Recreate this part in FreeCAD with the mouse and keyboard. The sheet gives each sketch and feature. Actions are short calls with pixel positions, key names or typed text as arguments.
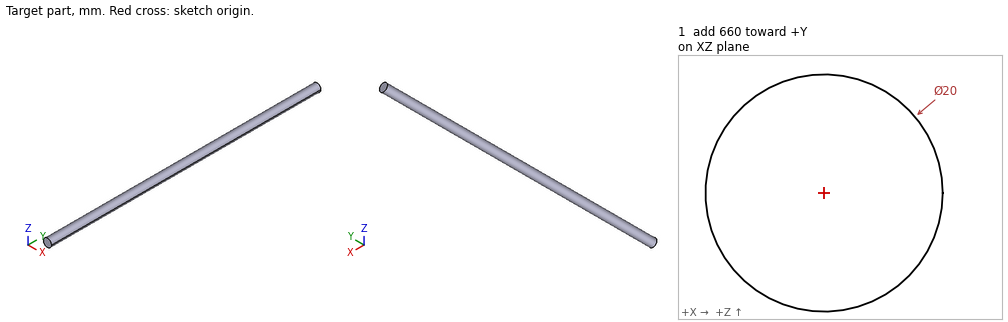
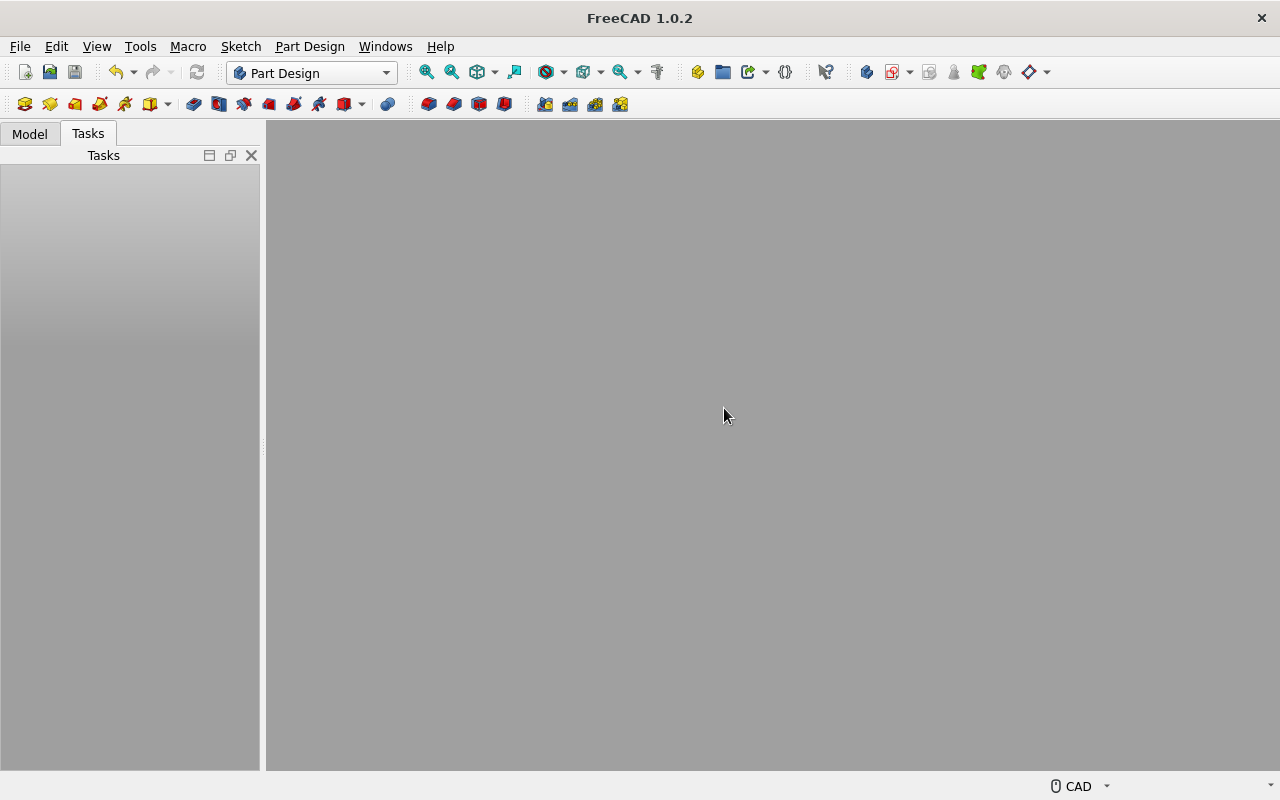
key(ctrl+n)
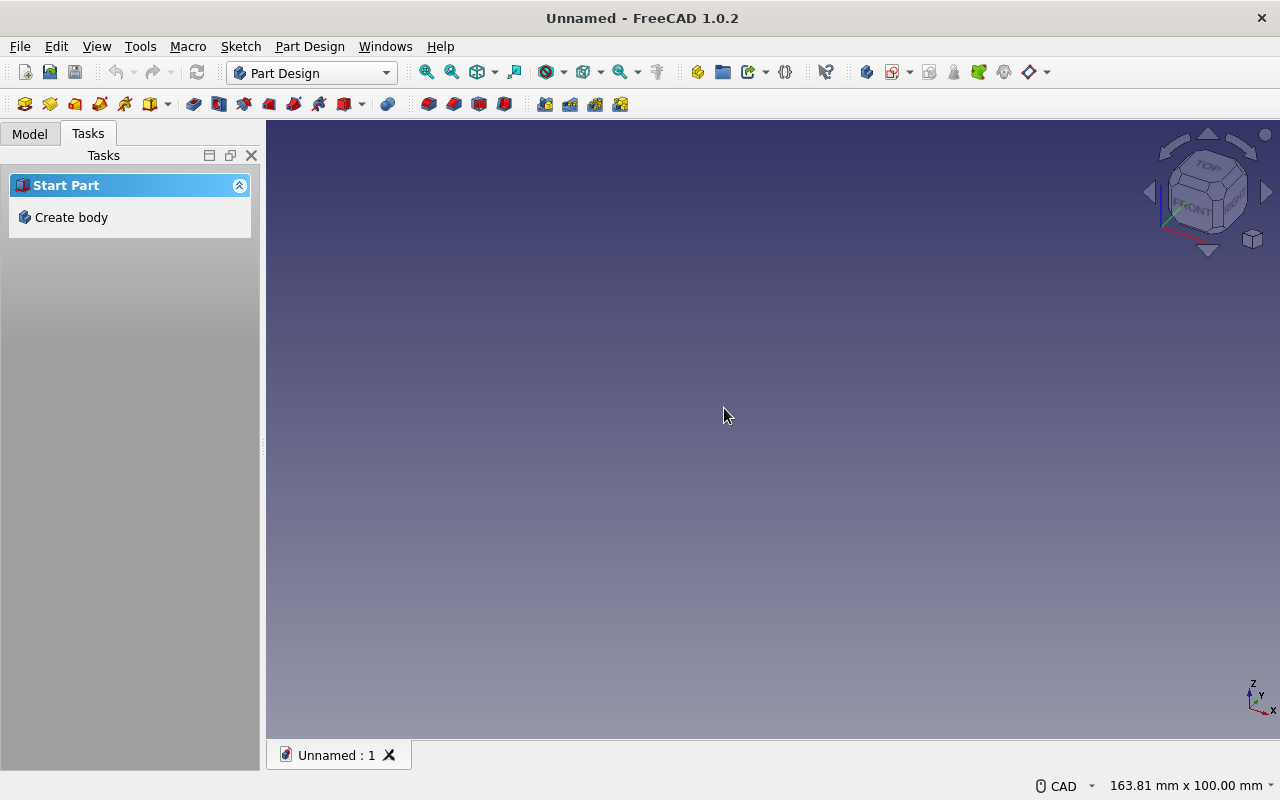
click(892, 72)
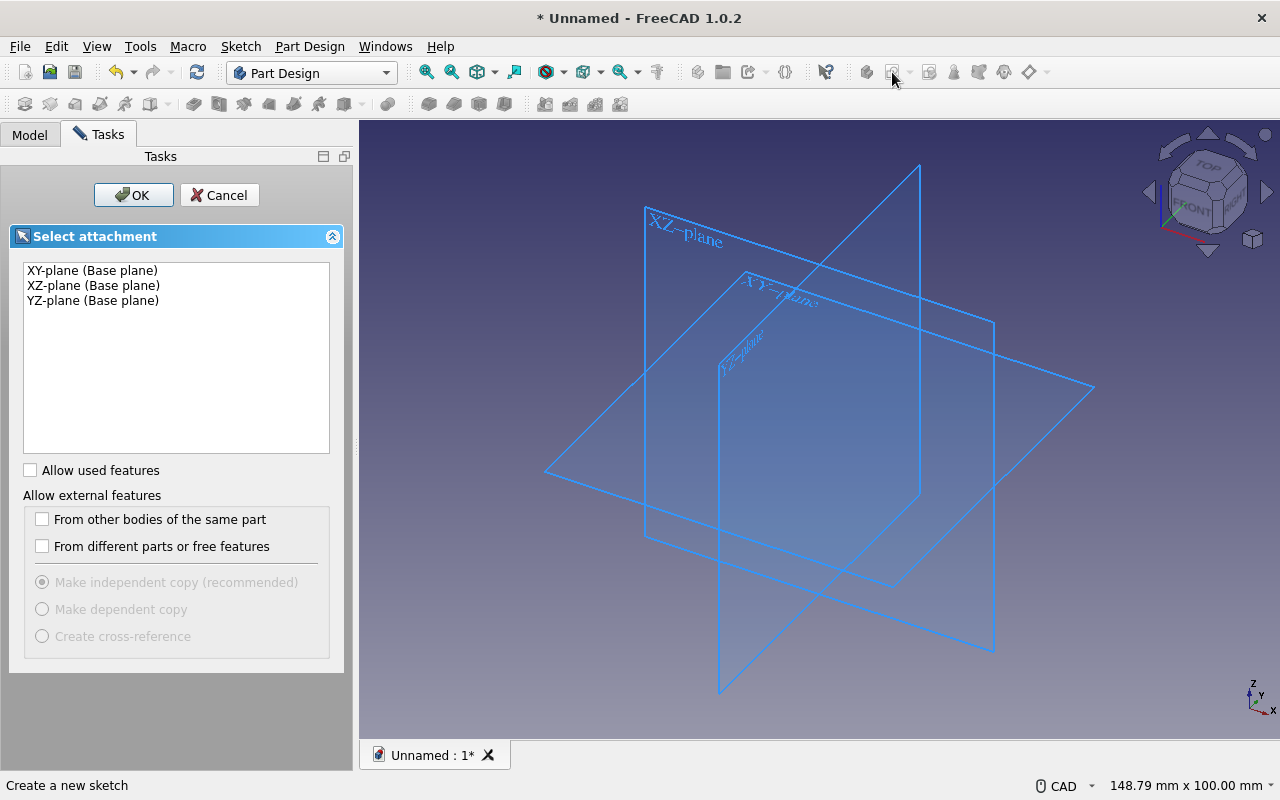
click(84, 286)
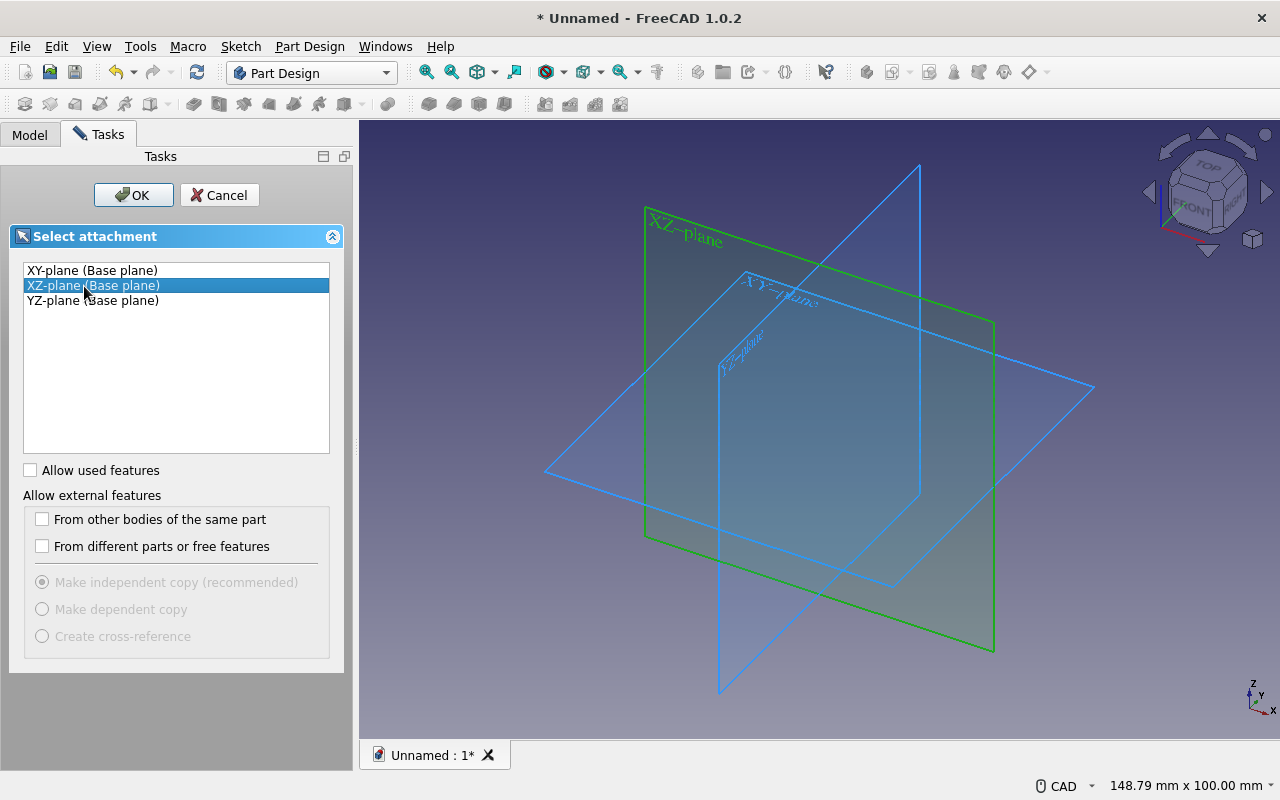
click(134, 195)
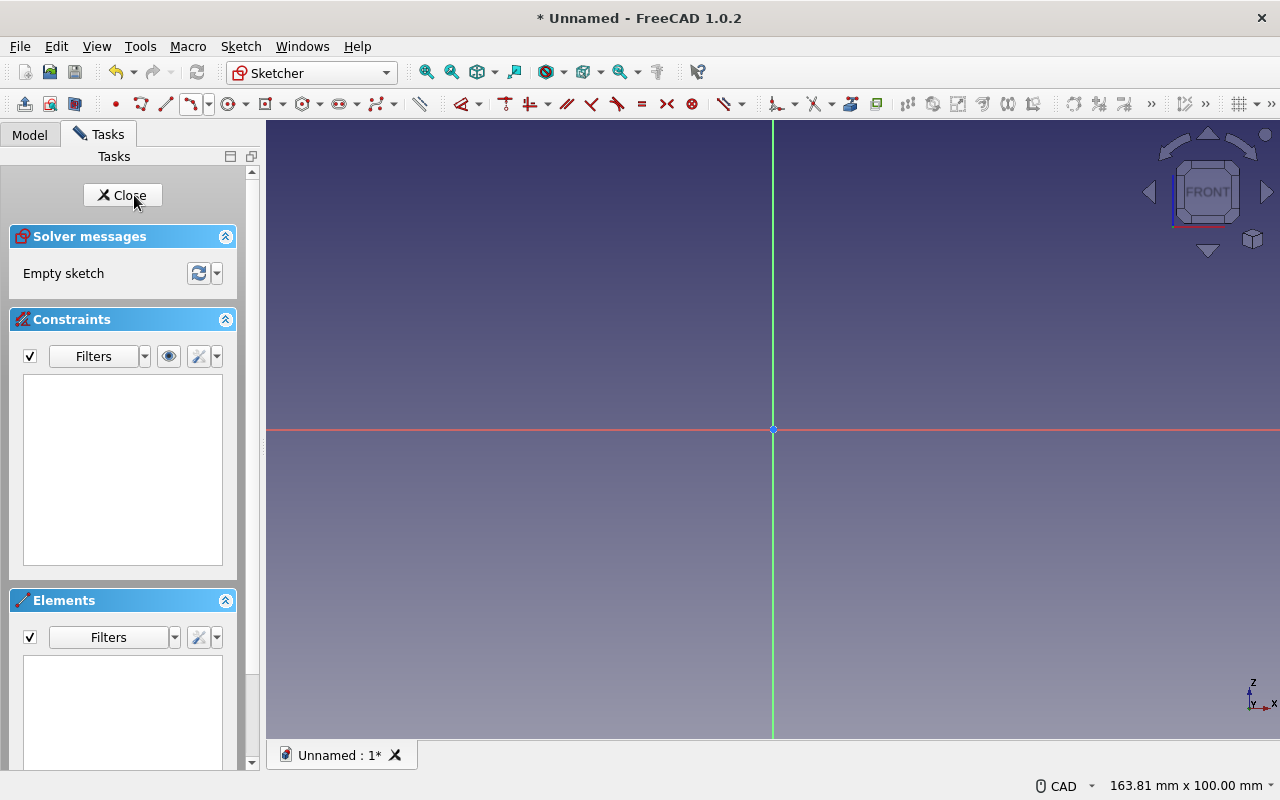
scroll(803, 430, up, 6)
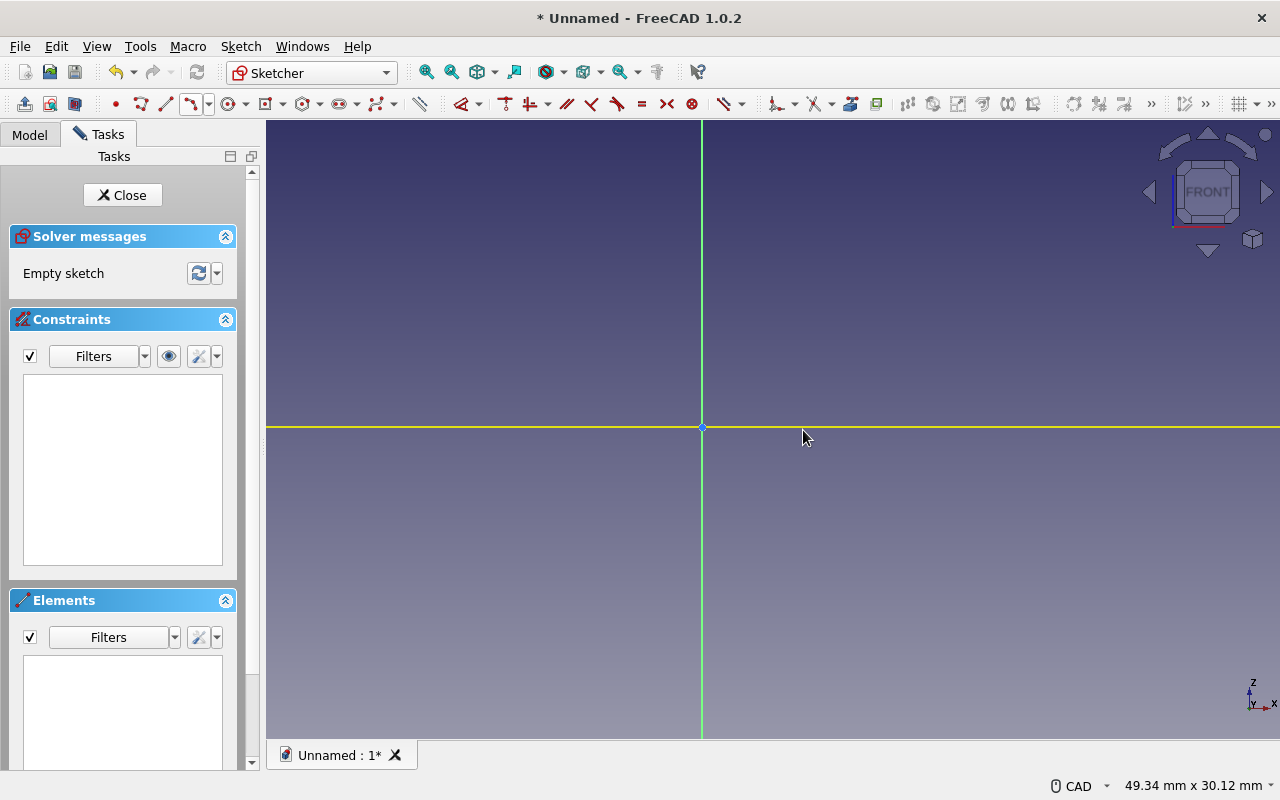
key(g)
key(c)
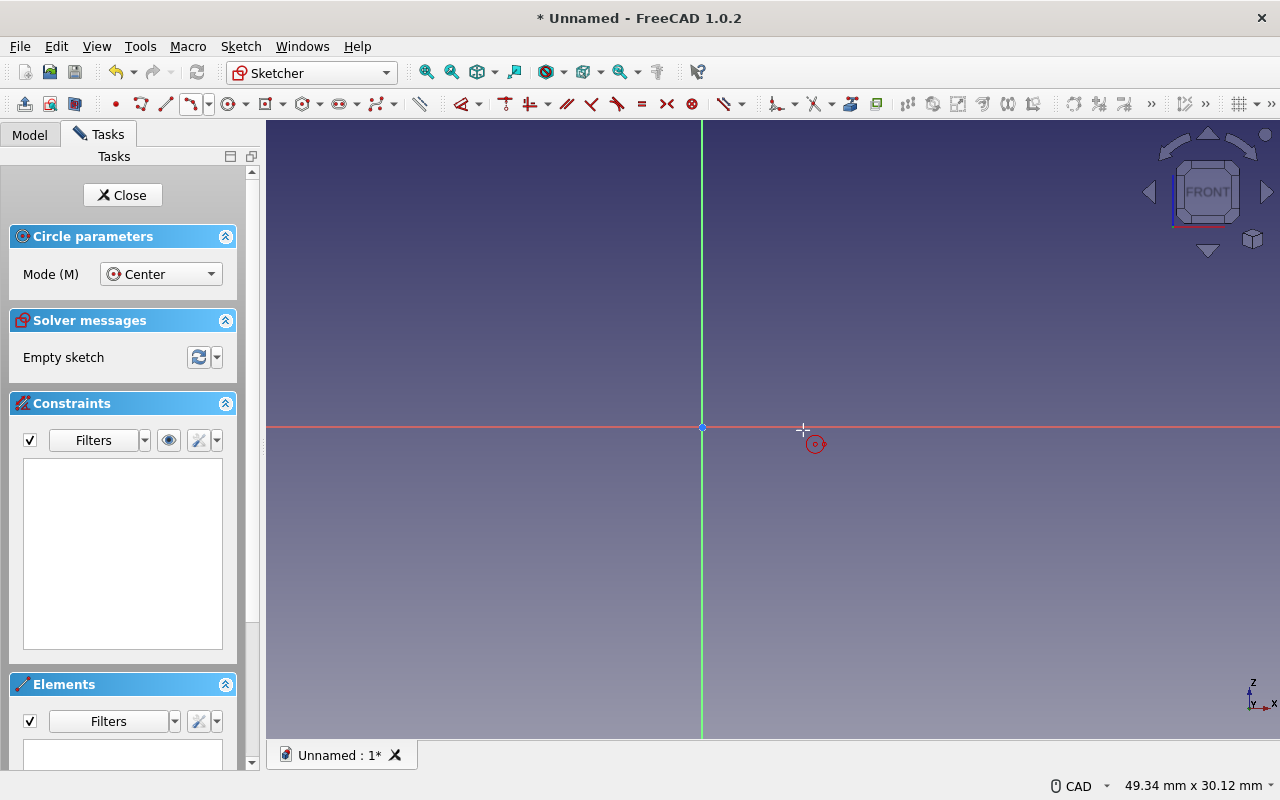
click(702, 427)
move(847, 282)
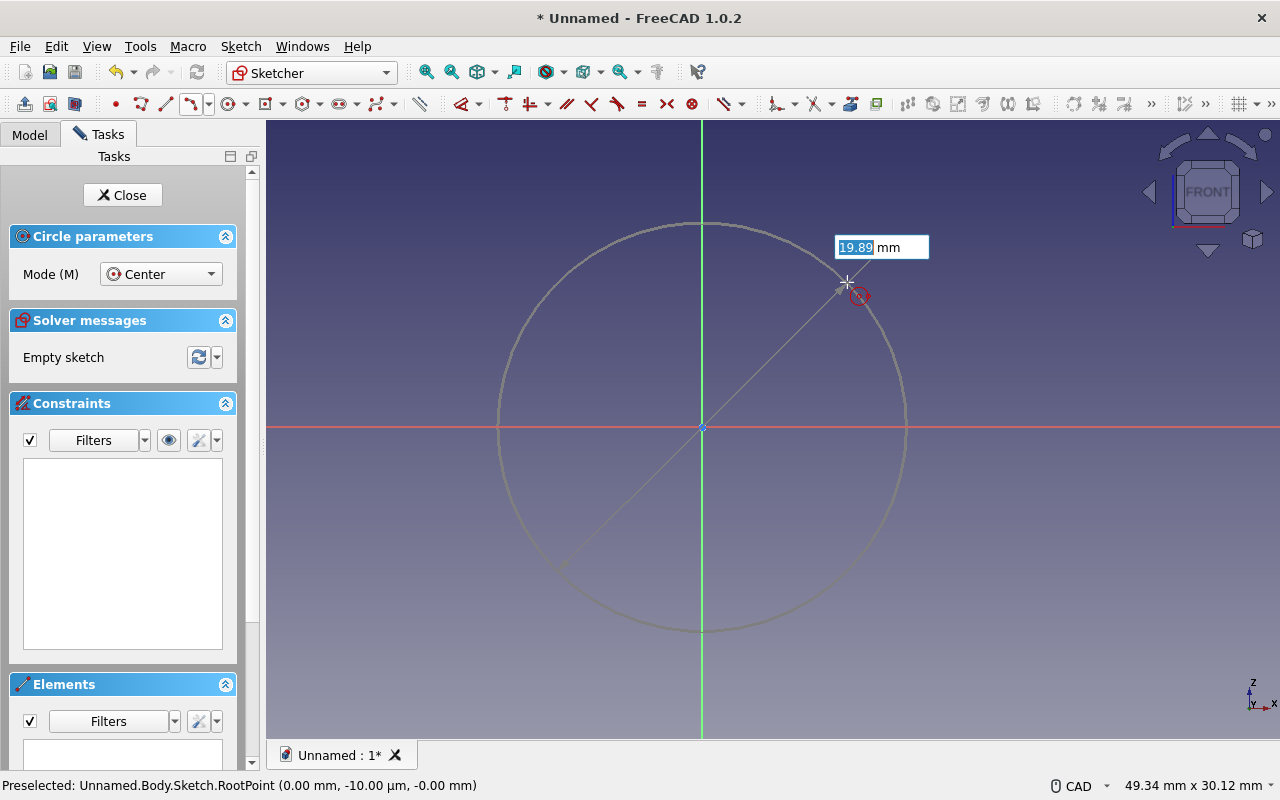
text(20)
key(Return)
key(Escape)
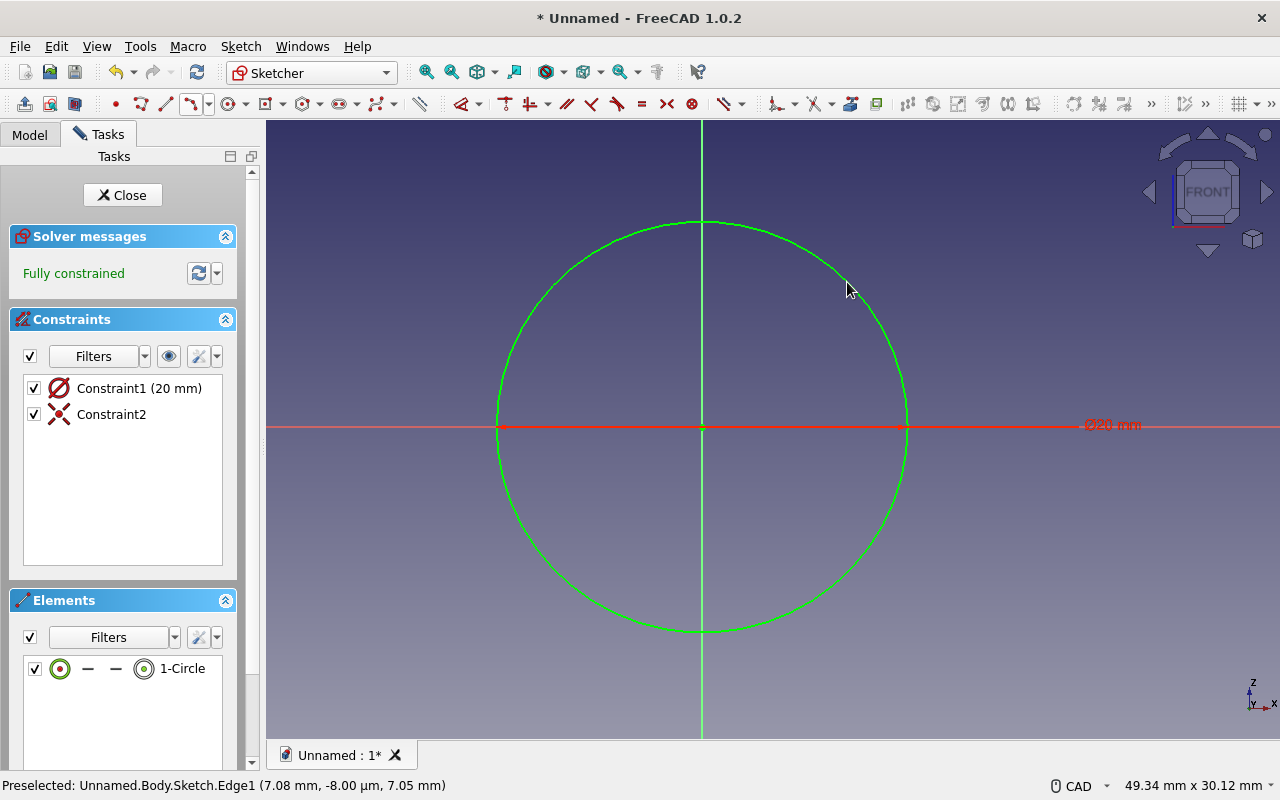
click(123, 195)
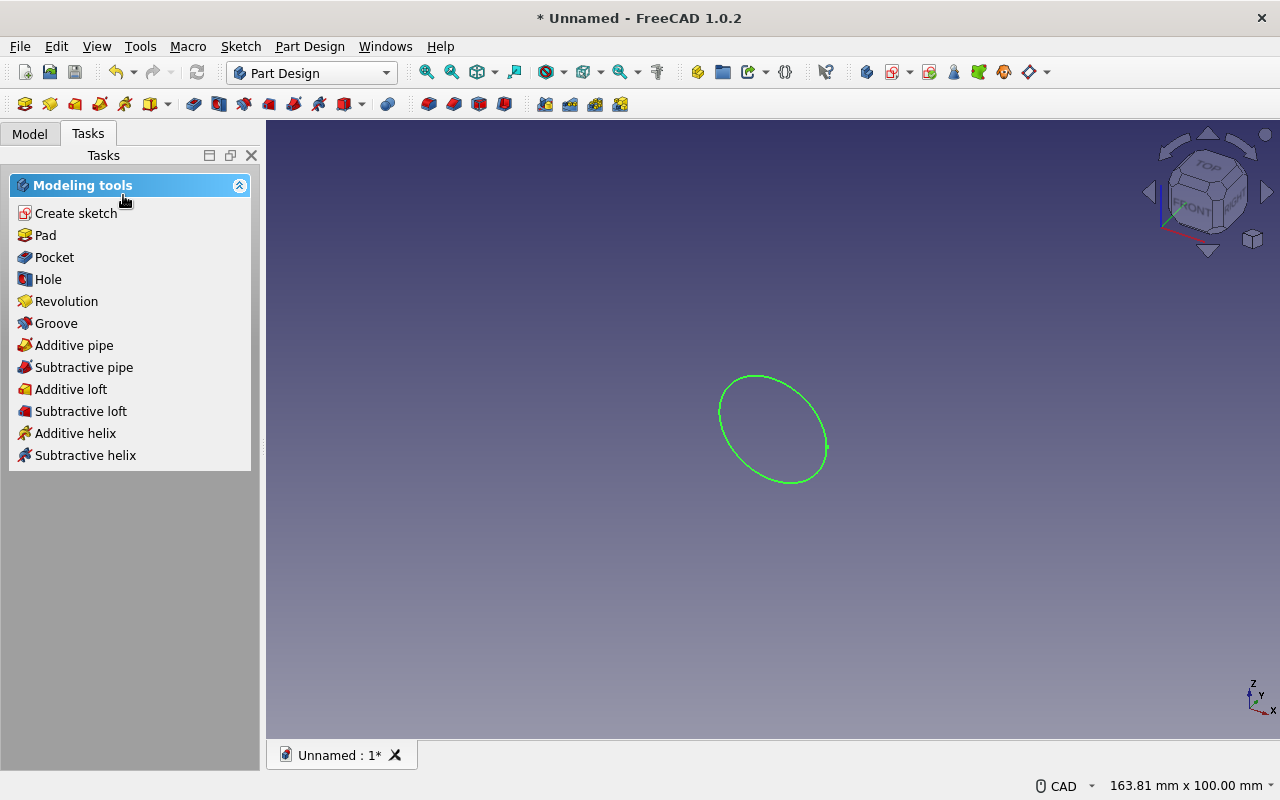
click(25, 104)